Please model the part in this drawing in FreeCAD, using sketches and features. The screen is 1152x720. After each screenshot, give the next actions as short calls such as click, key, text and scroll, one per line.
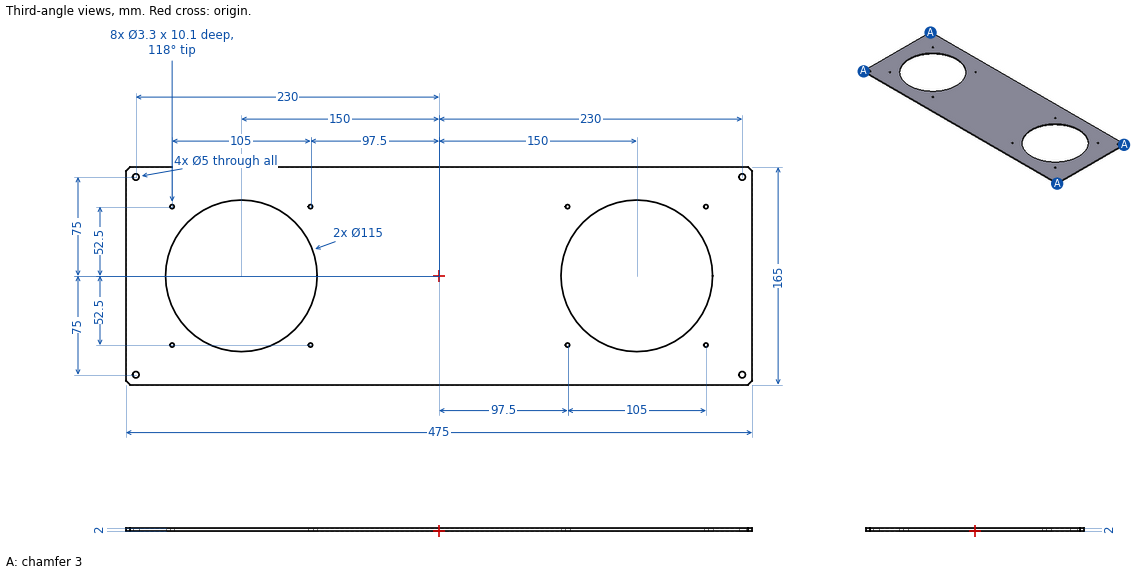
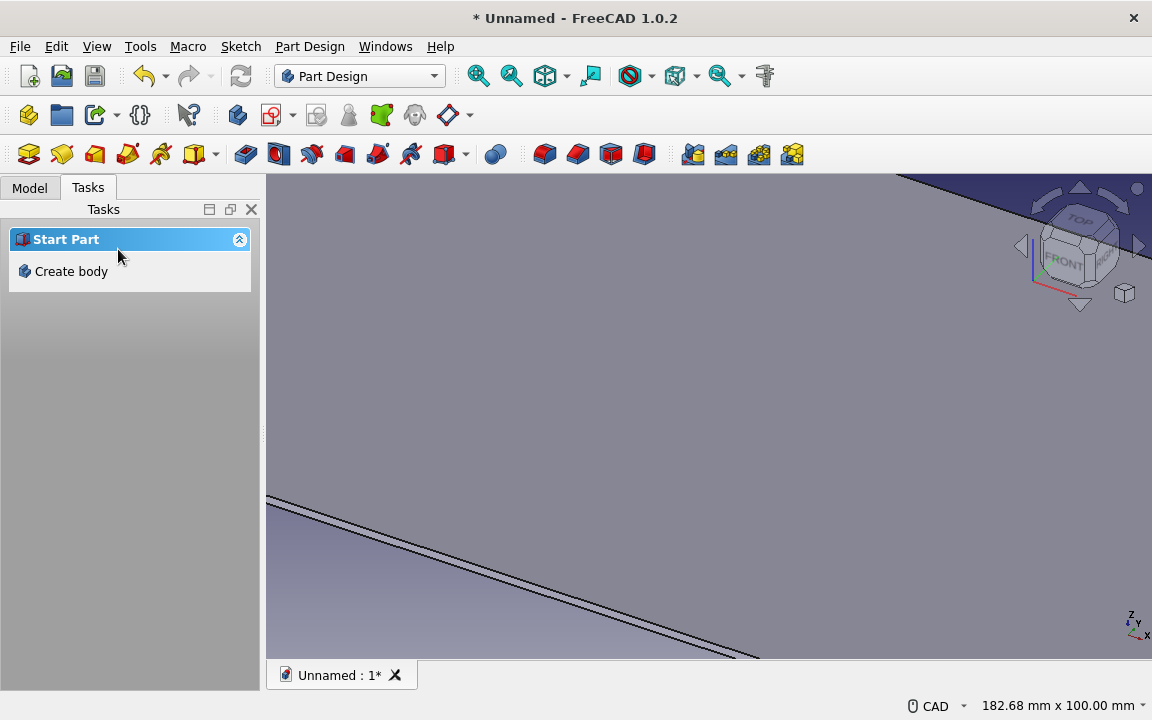
key(v)
key(f)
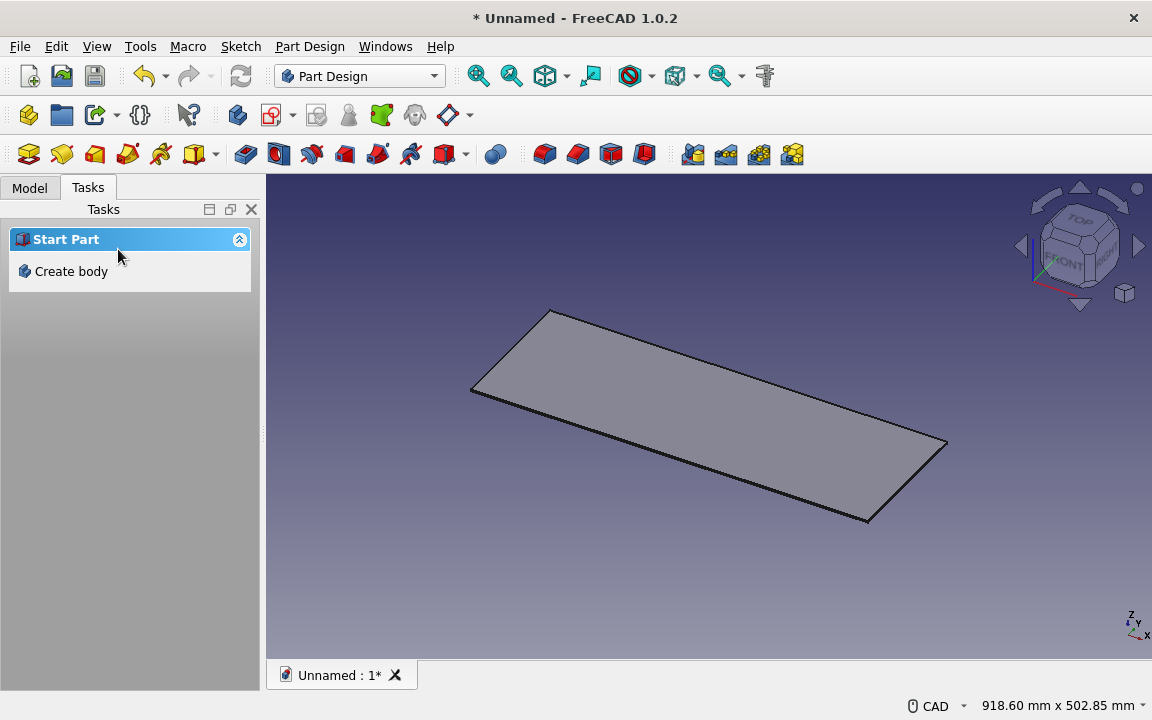
click(822, 452)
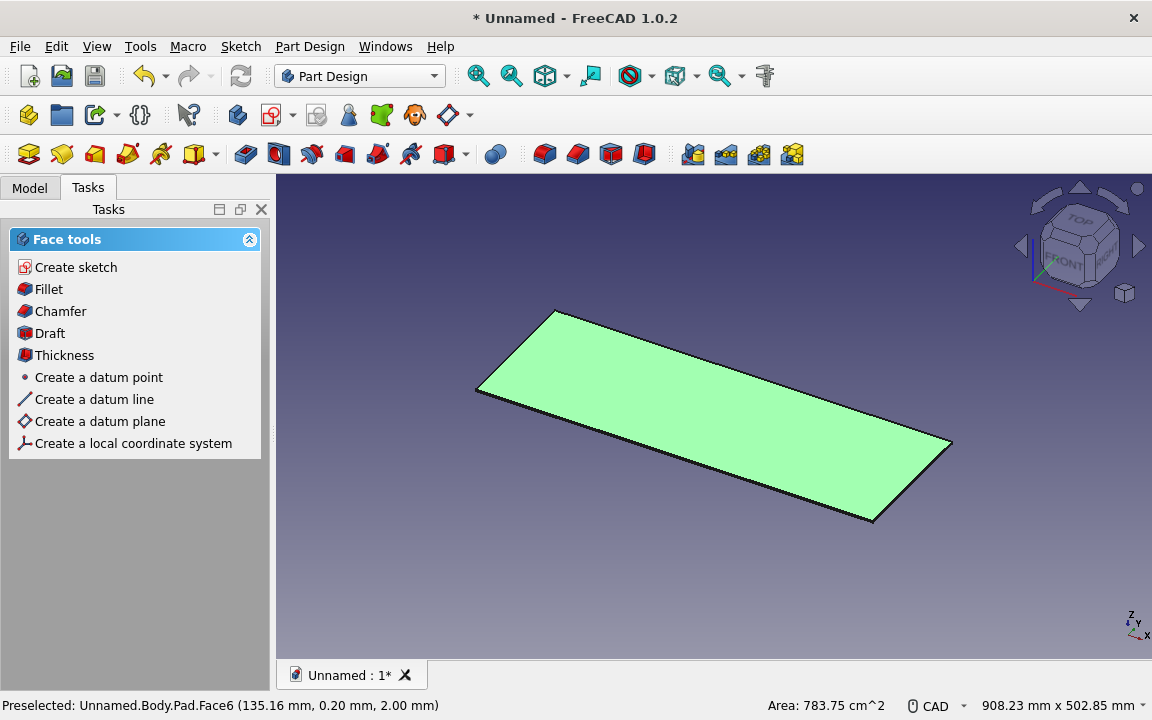
click(270, 116)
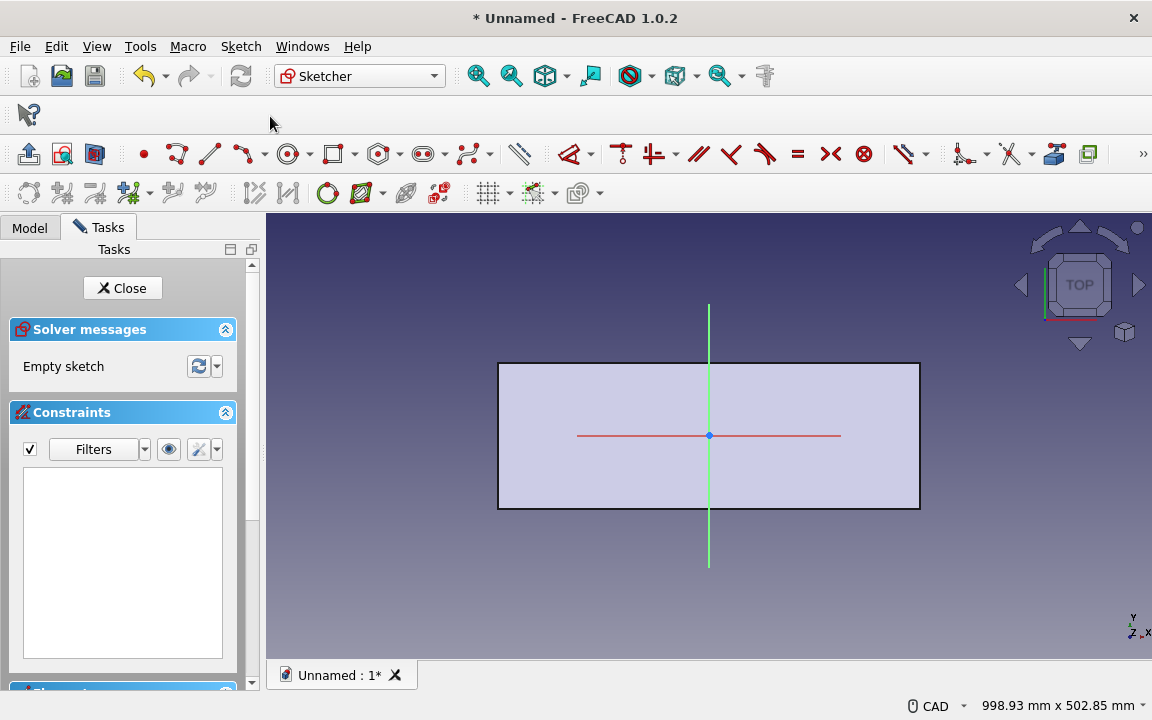
click(288, 154)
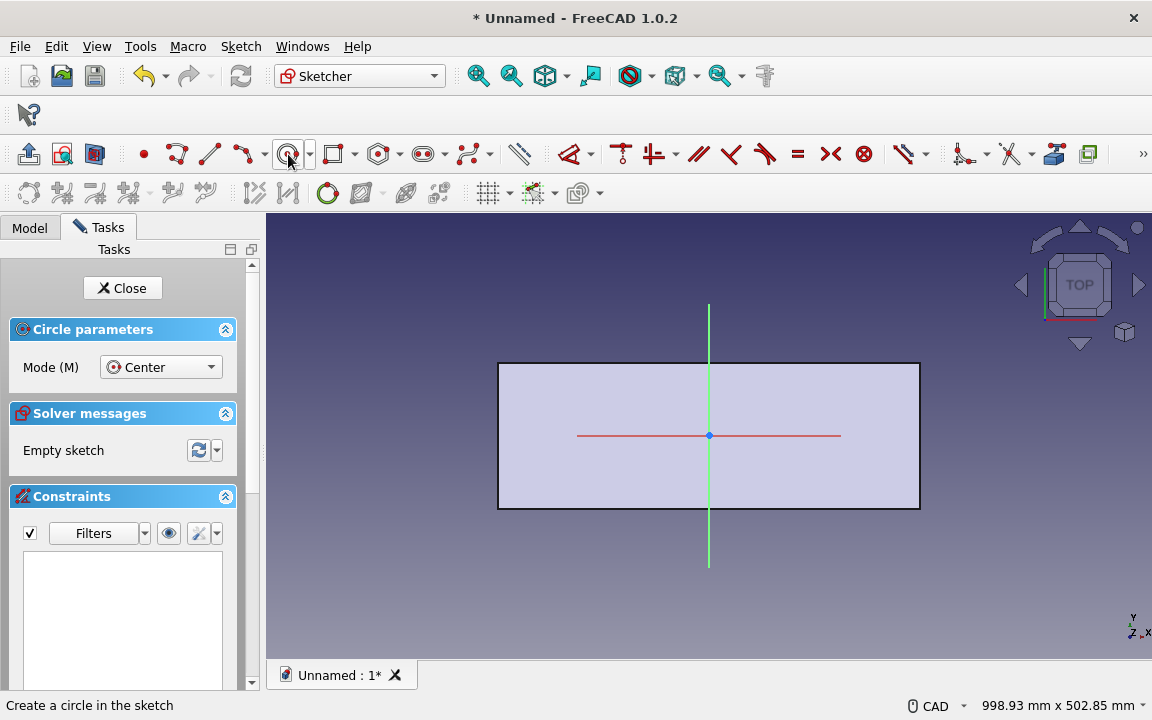
scroll(505, 369, up, 12)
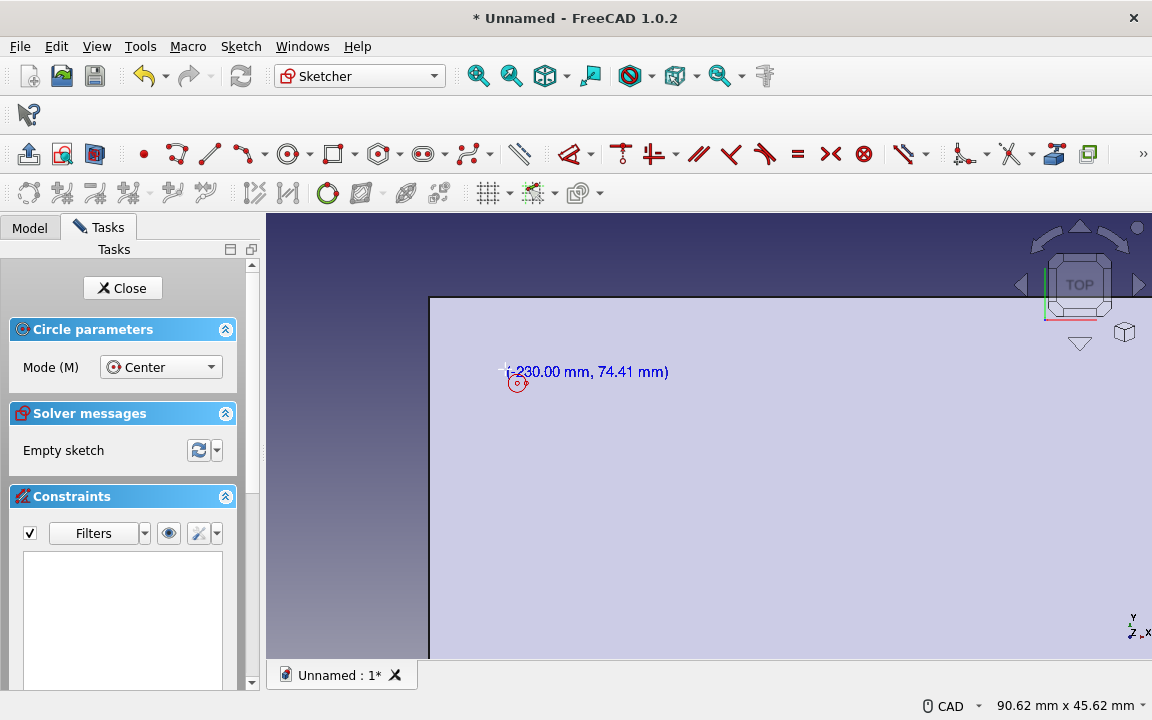
scroll(378, 353, down, 11)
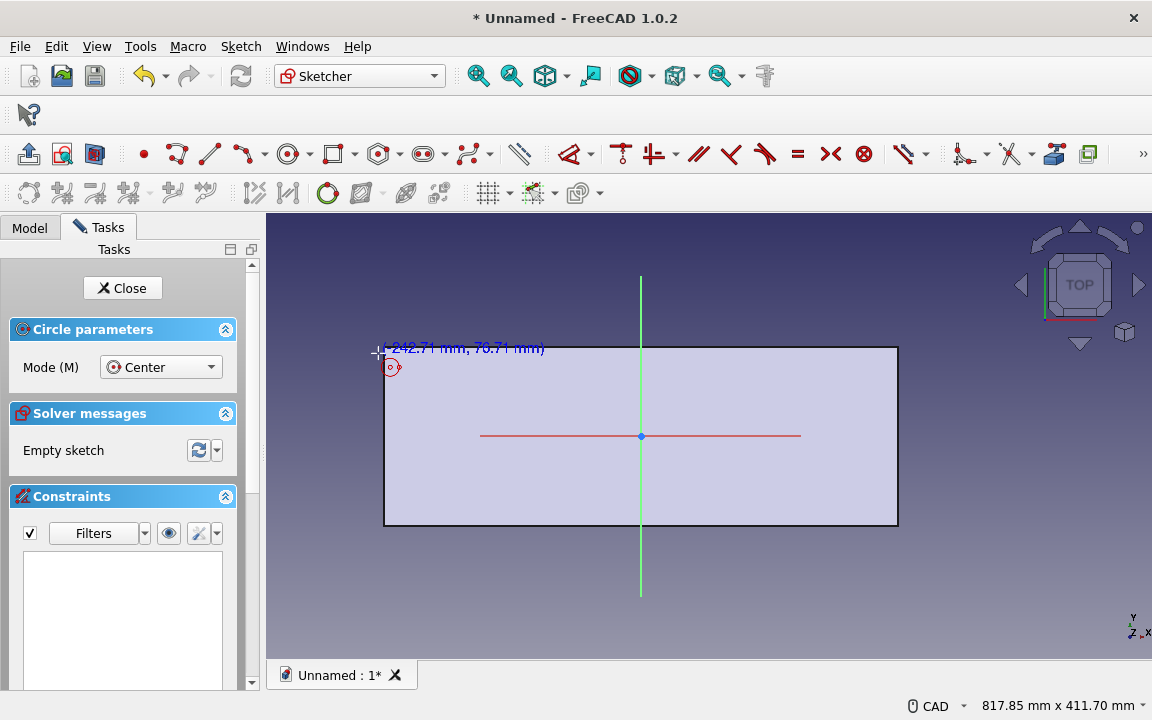
click(392, 355)
move(394, 353)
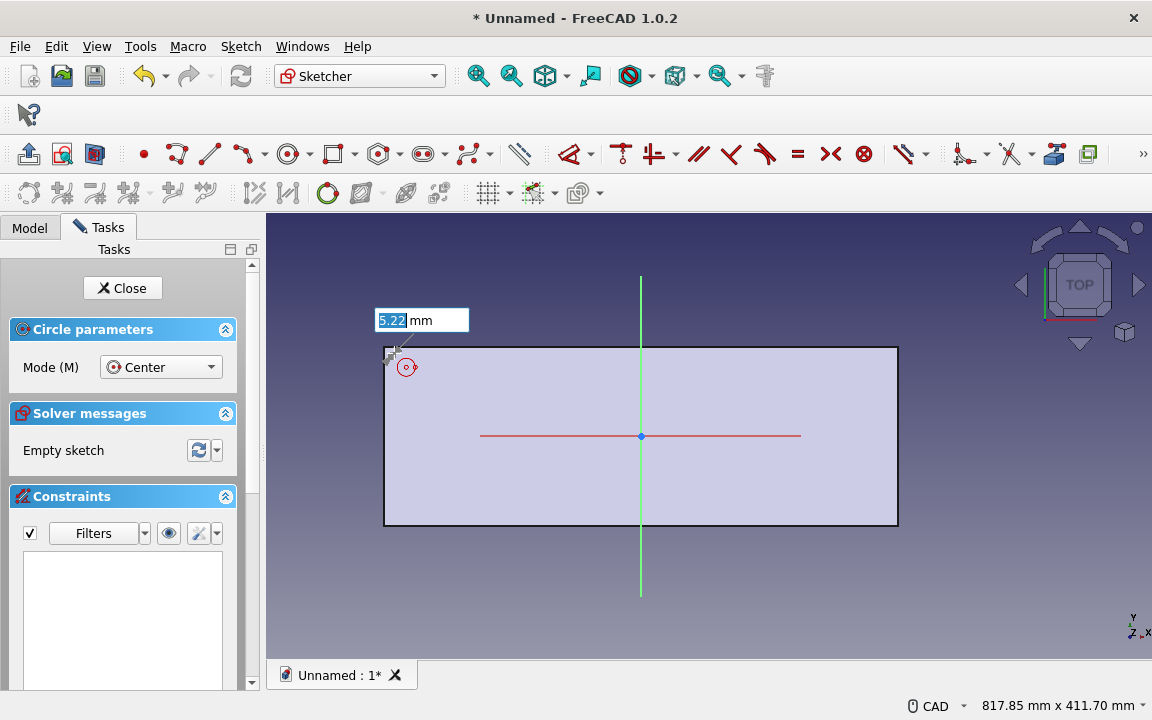
text(5)
key(Return)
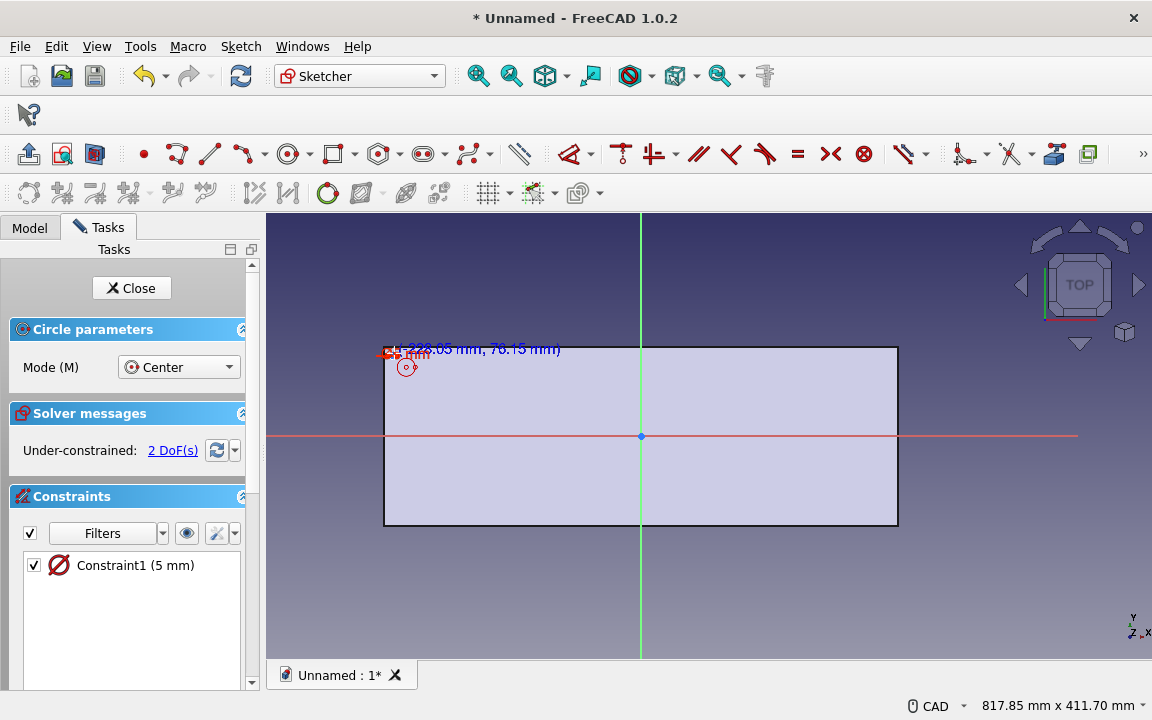
scroll(392, 518, up, 11)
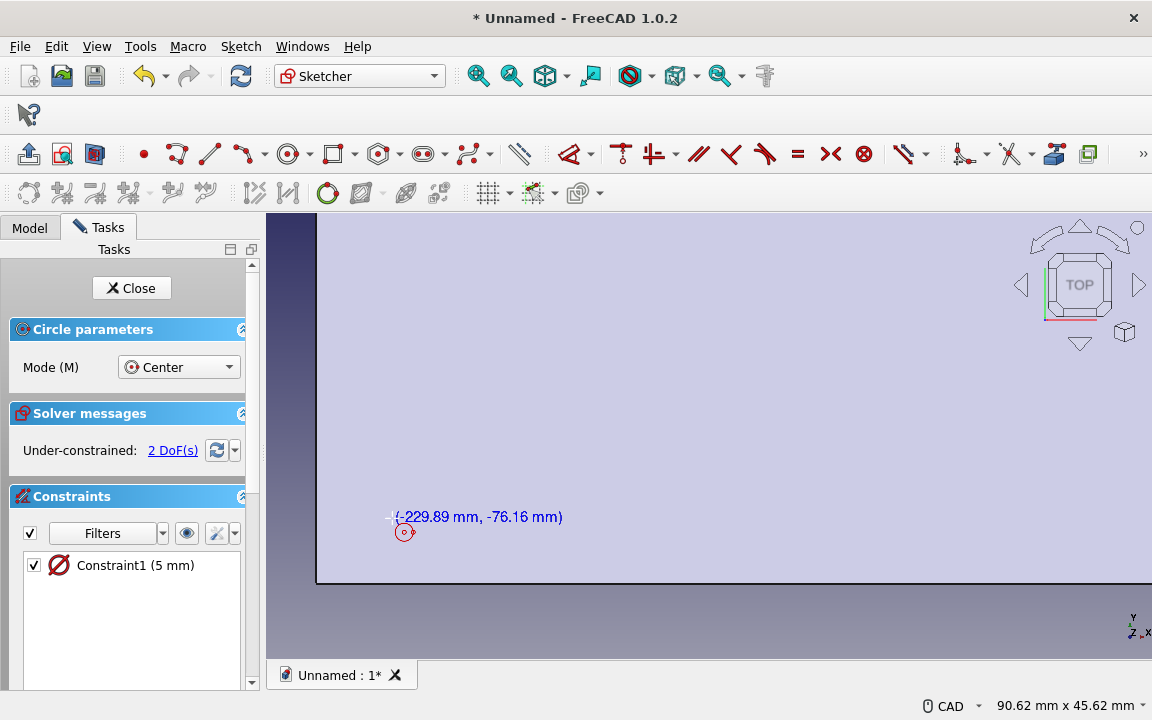
scroll(392, 518, down, 11)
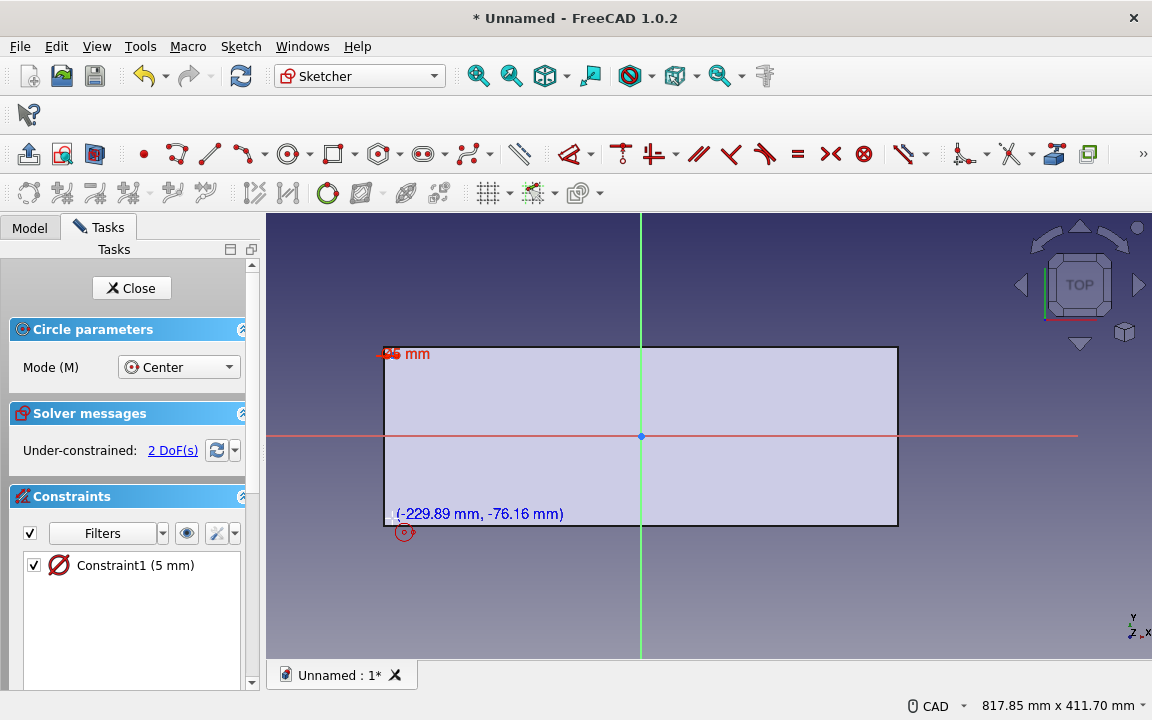
click(392, 518)
move(394, 516)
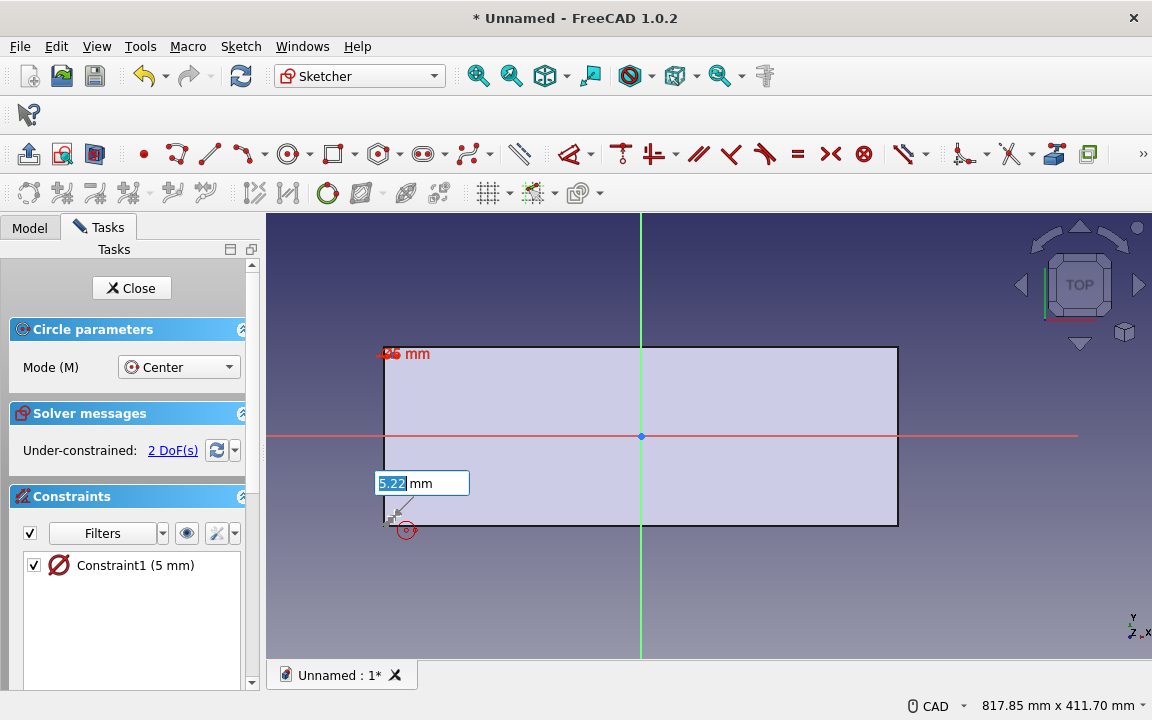
text(5)
key(Return)